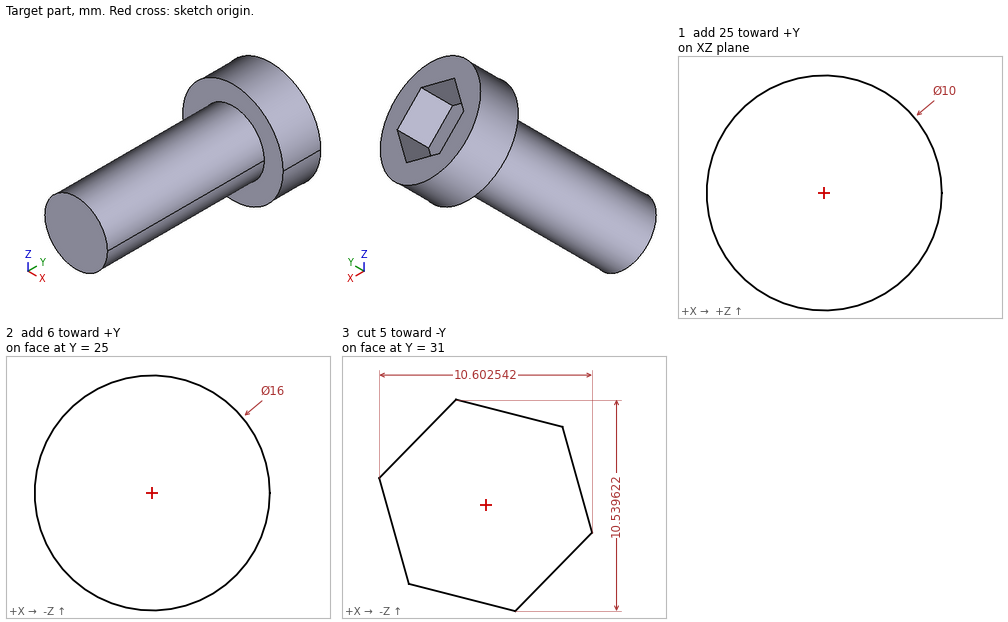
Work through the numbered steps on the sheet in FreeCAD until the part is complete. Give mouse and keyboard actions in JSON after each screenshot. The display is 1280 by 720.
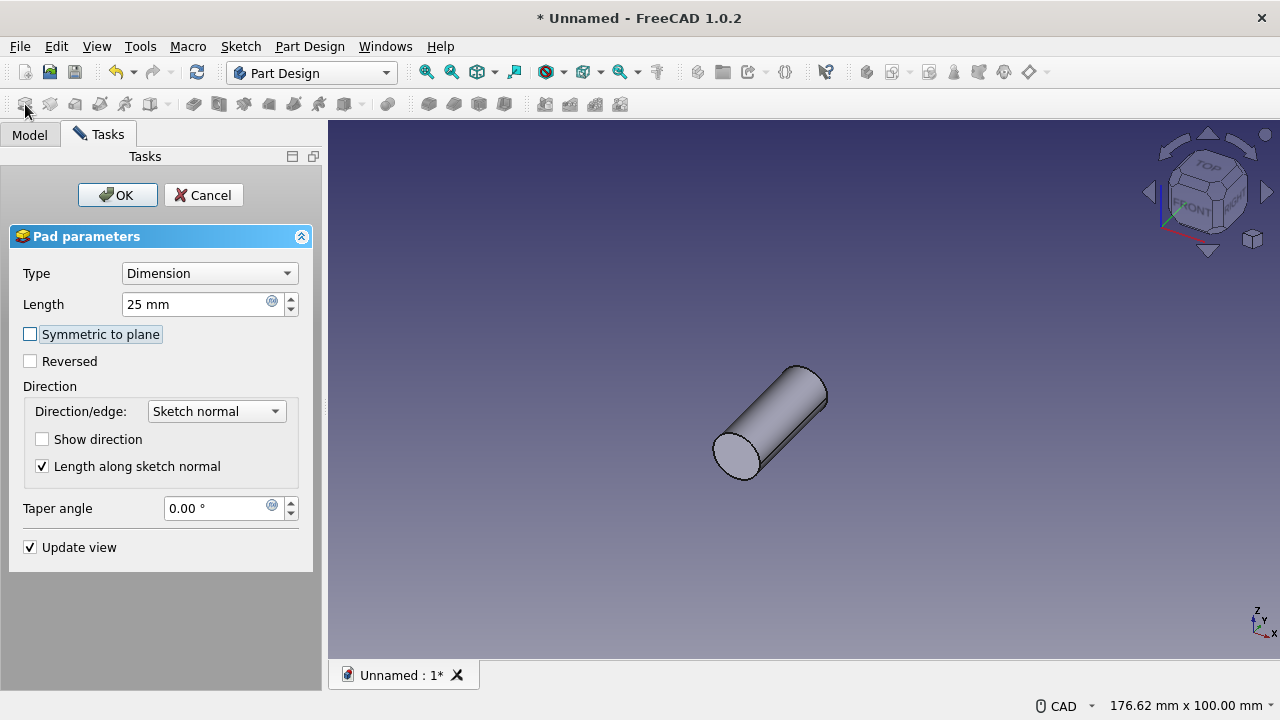
{"action": "left_click", "coordinate": [31, 361]}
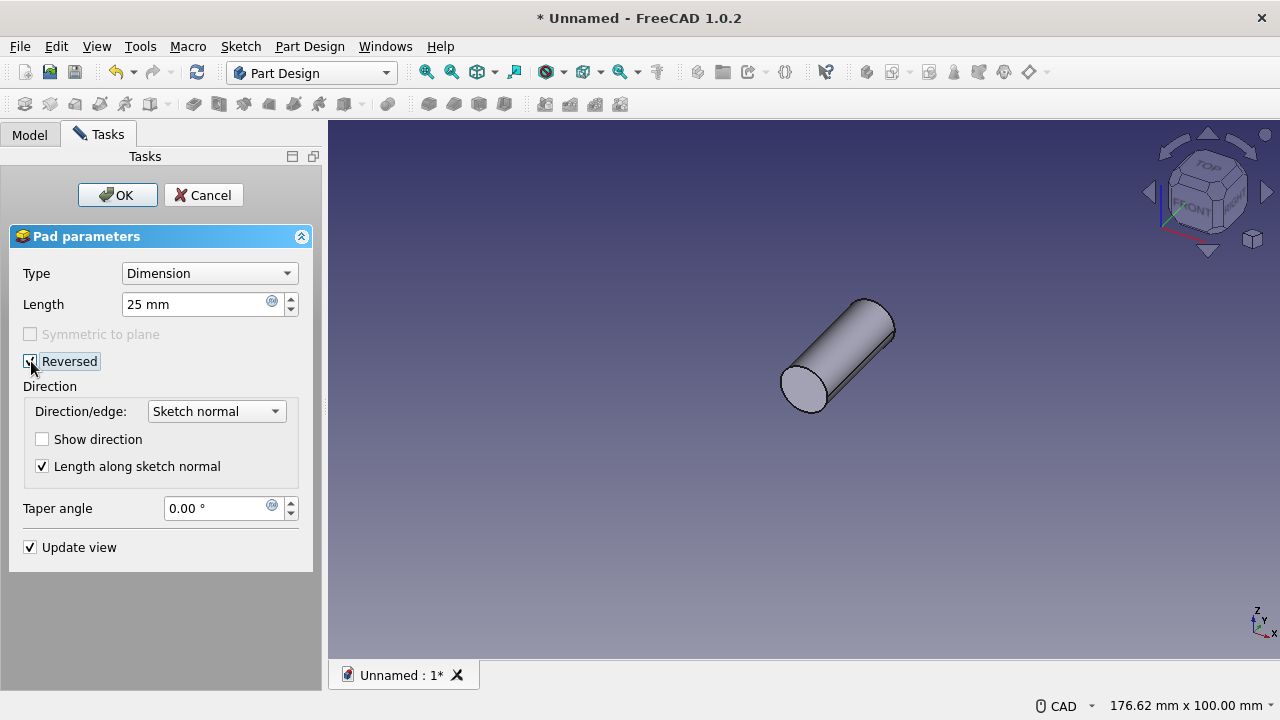
{"action": "left_click", "coordinate": [118, 195]}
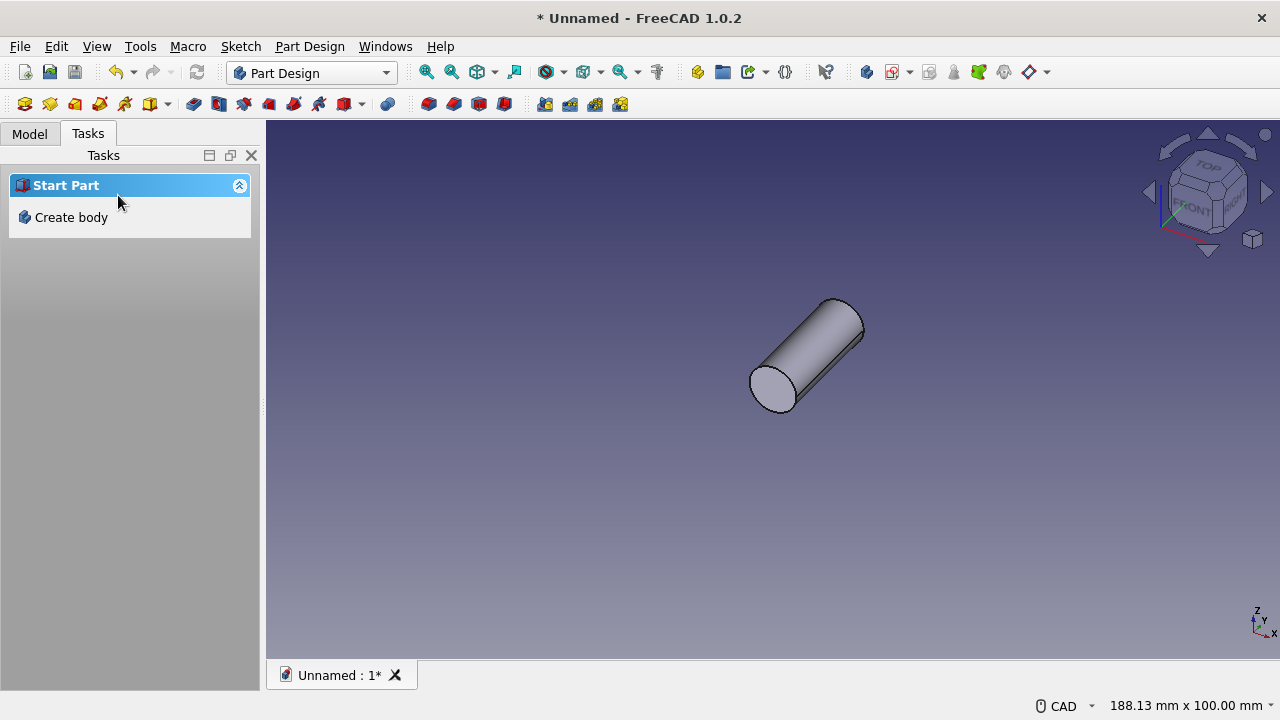
{"action": "left_click", "coordinate": [427, 72]}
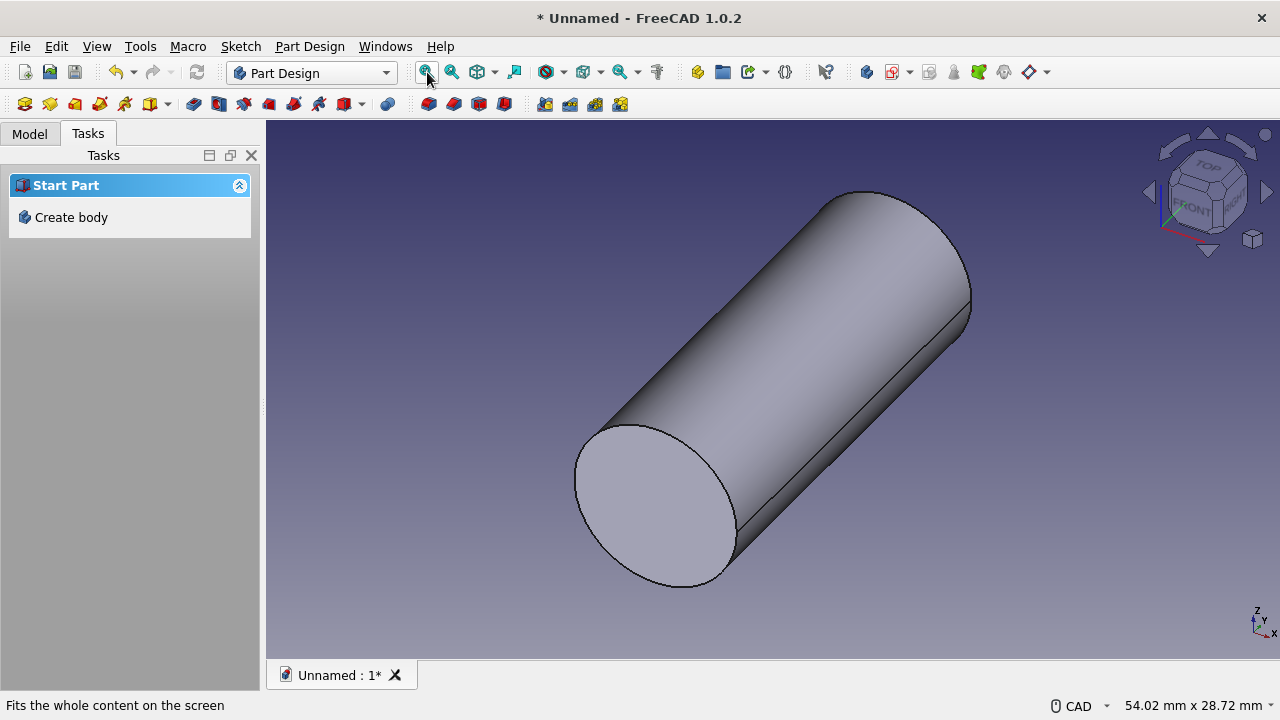
{"action": "key", "text": "4"}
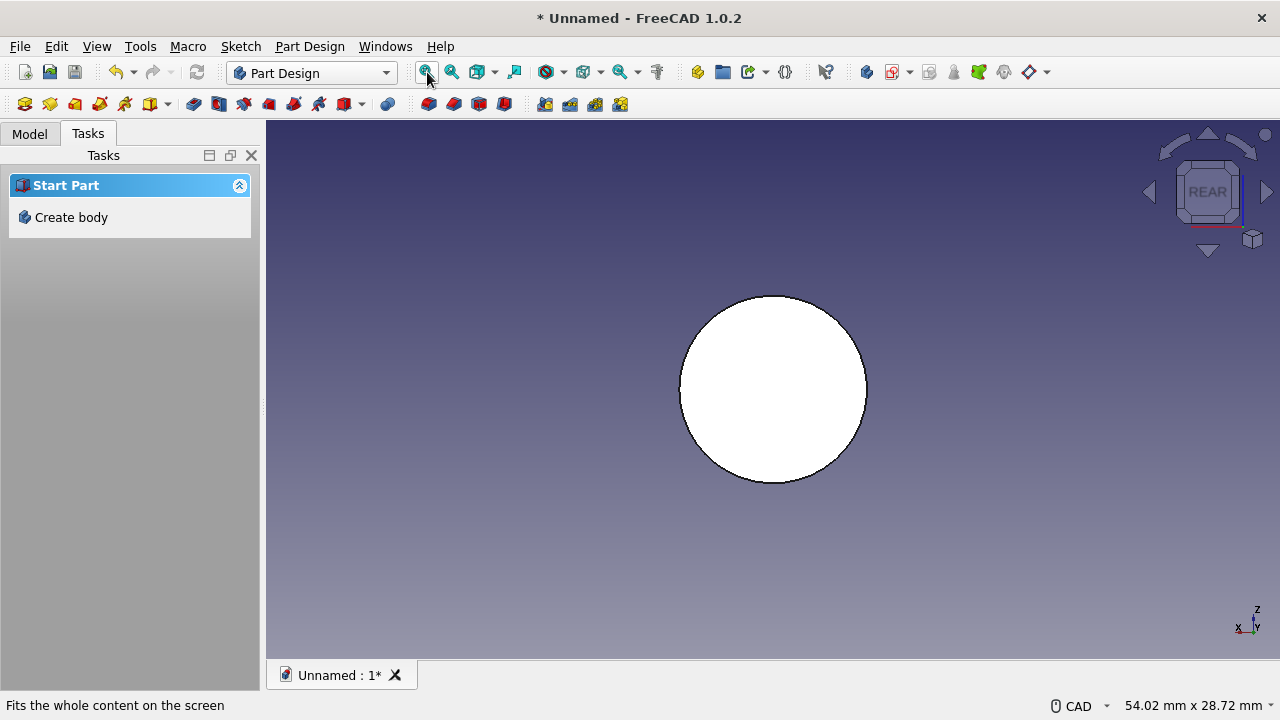
{"action": "key", "text": "v f"}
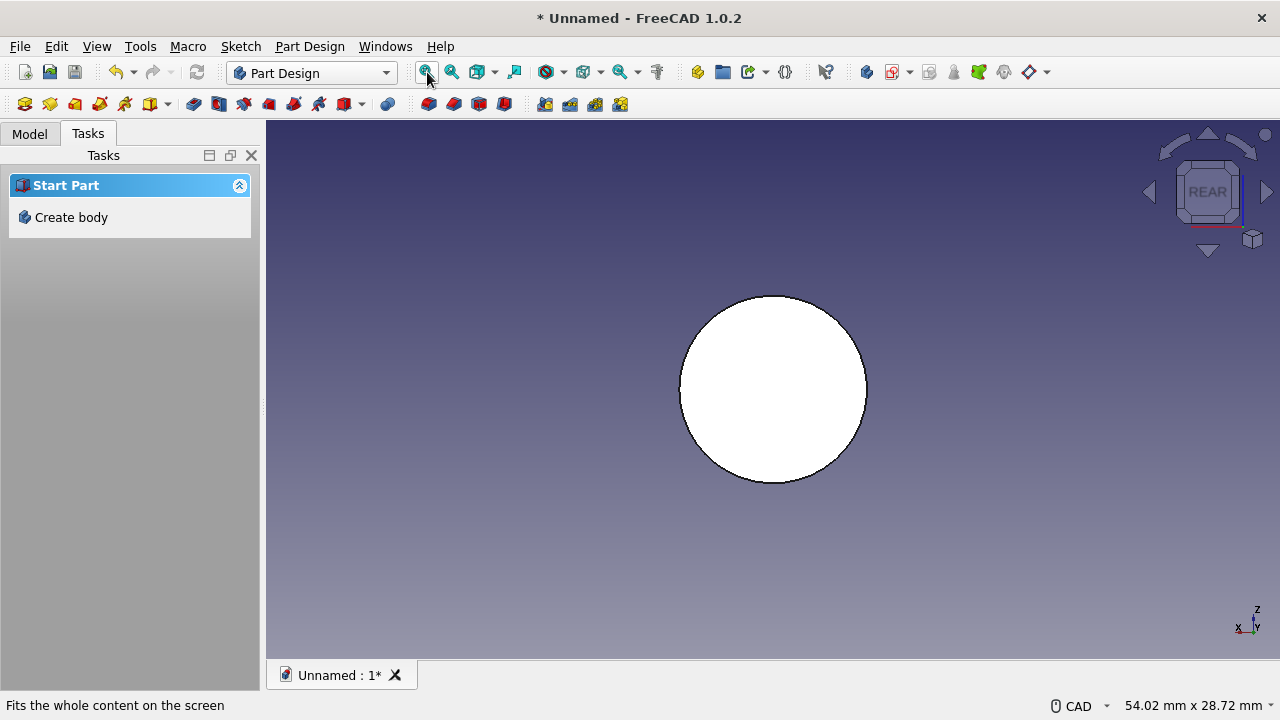
{"action": "left_click", "coordinate": [773, 389]}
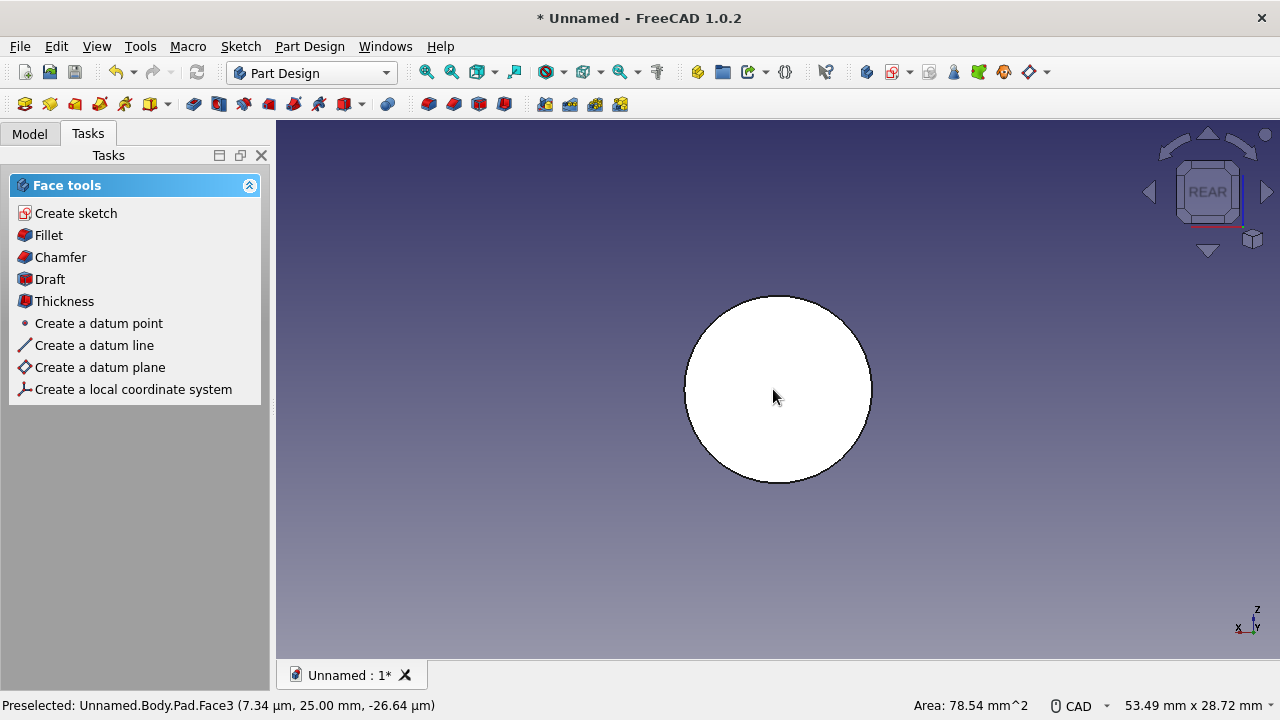
{"action": "left_click", "coordinate": [892, 72]}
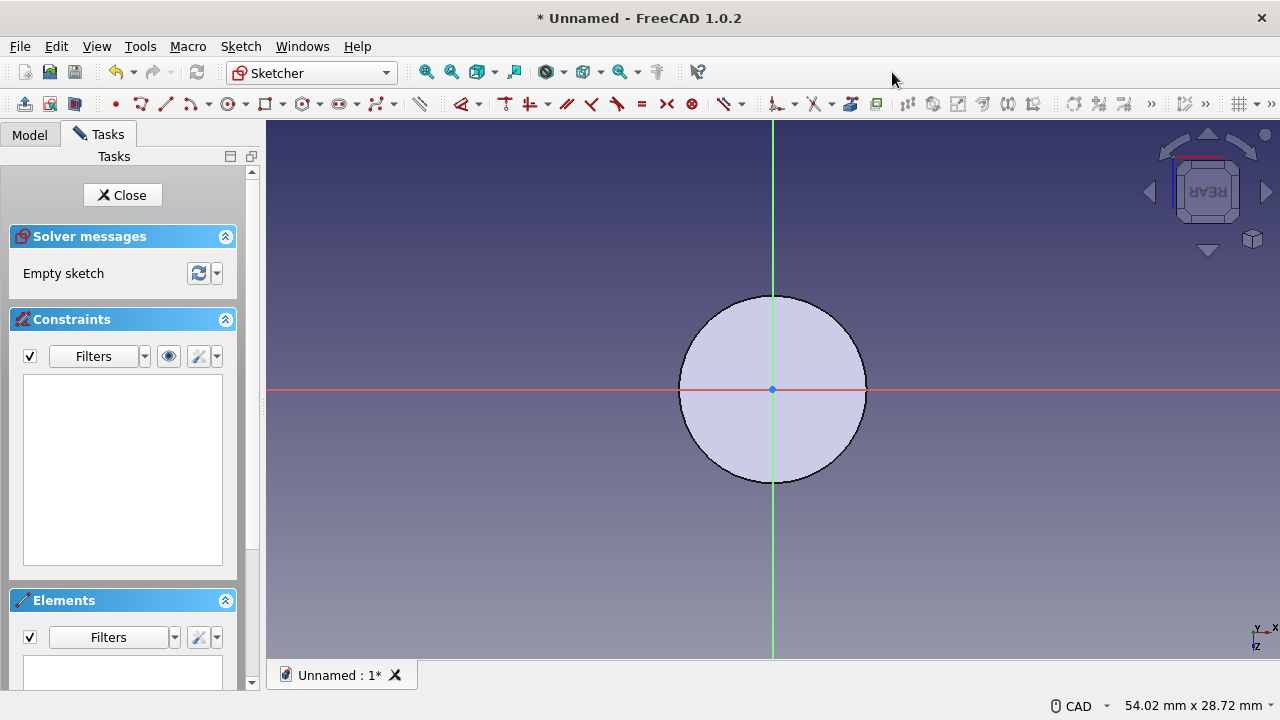
{"action": "key", "text": "g c"}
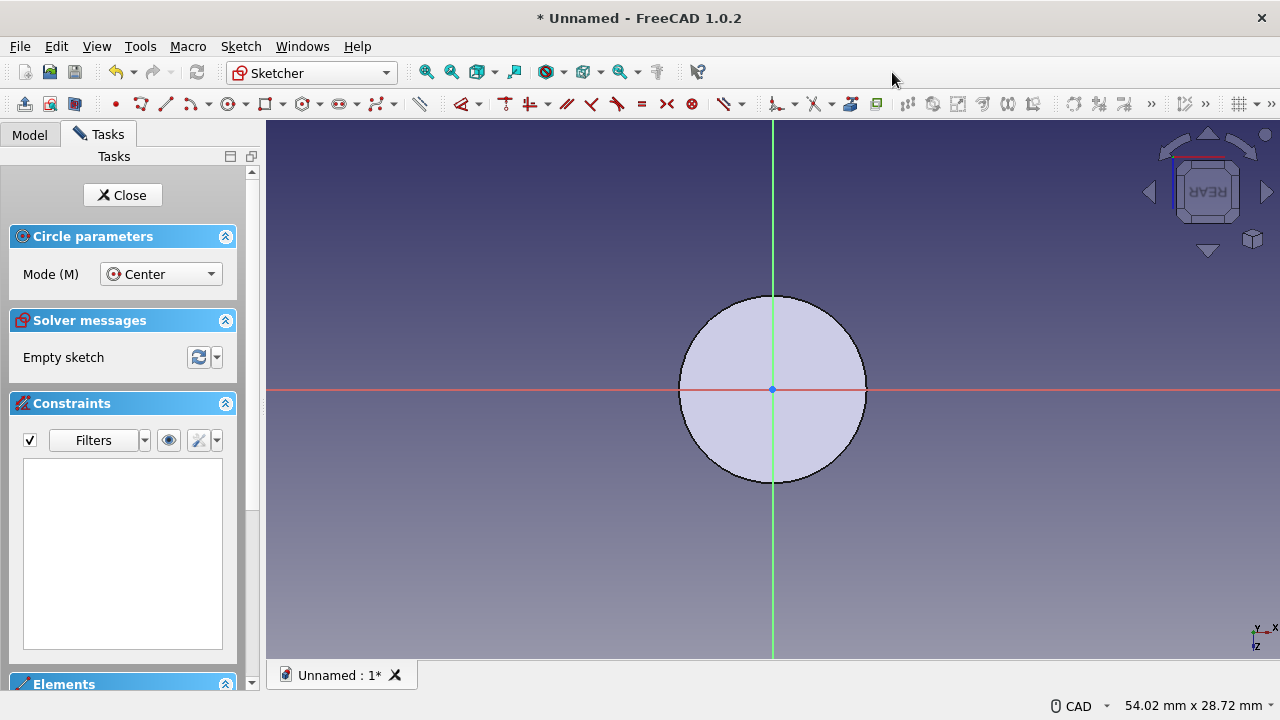
{"action": "left_click", "coordinate": [773, 389]}
{"action": "mouse_move", "coordinate": [879, 283]}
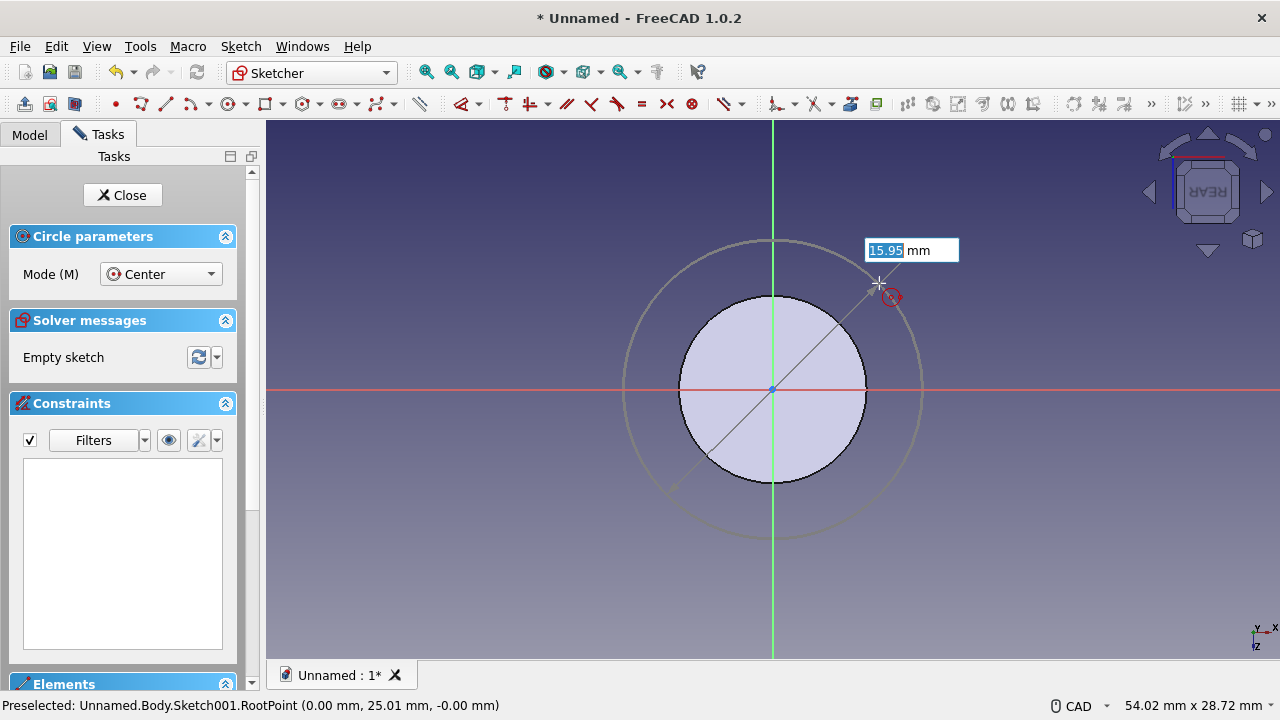
{"action": "type", "text": "16"}
{"action": "key", "text": "Return"}
{"action": "key", "text": "Escape"}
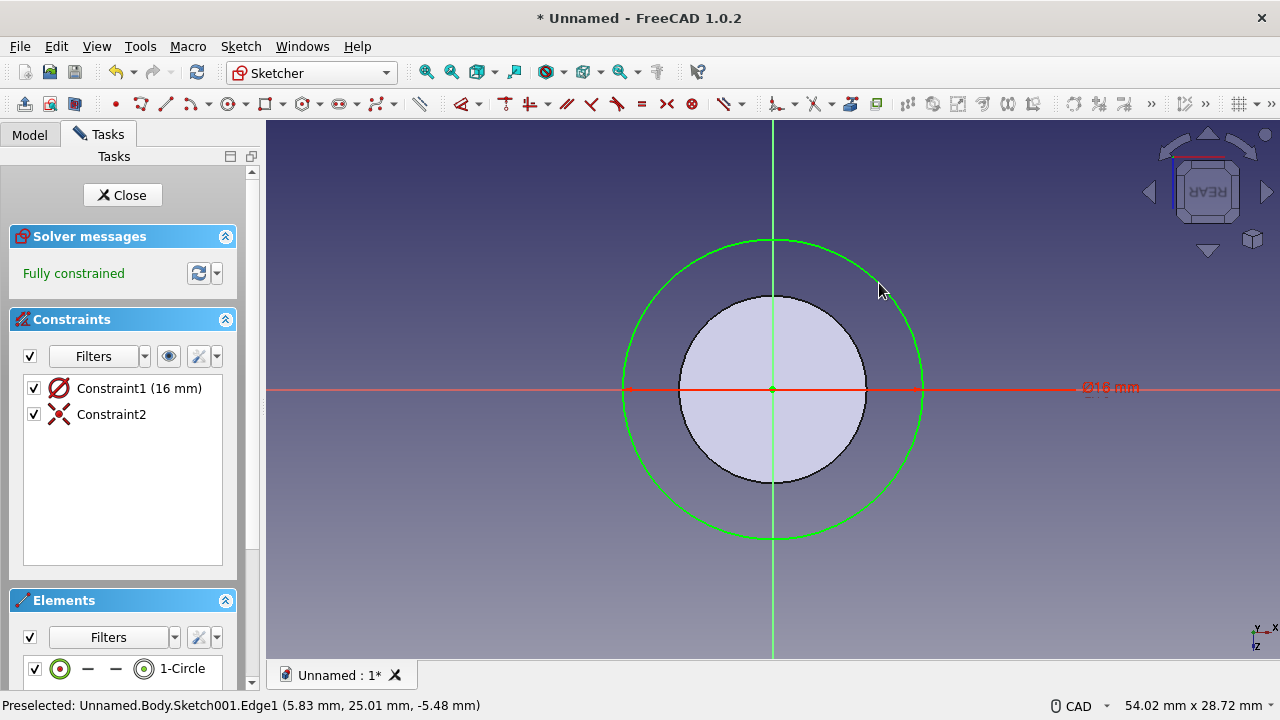
{"action": "left_click", "coordinate": [123, 195]}